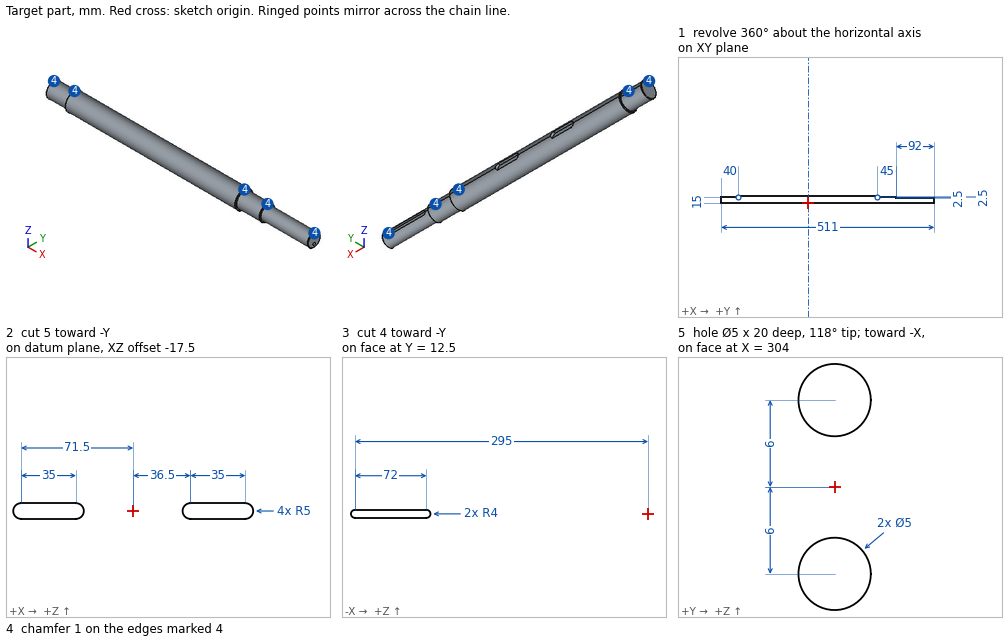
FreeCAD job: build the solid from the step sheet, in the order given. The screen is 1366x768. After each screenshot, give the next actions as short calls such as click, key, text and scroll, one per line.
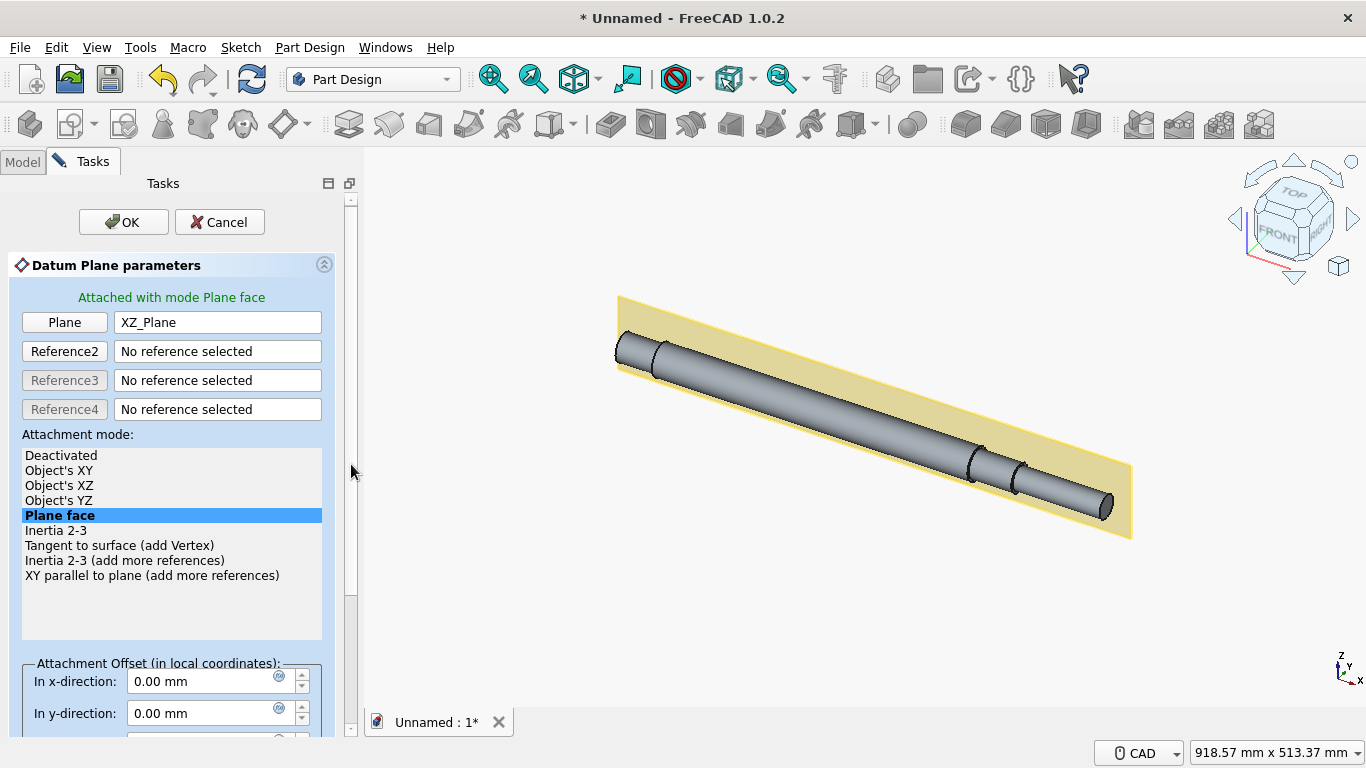
click(124, 222)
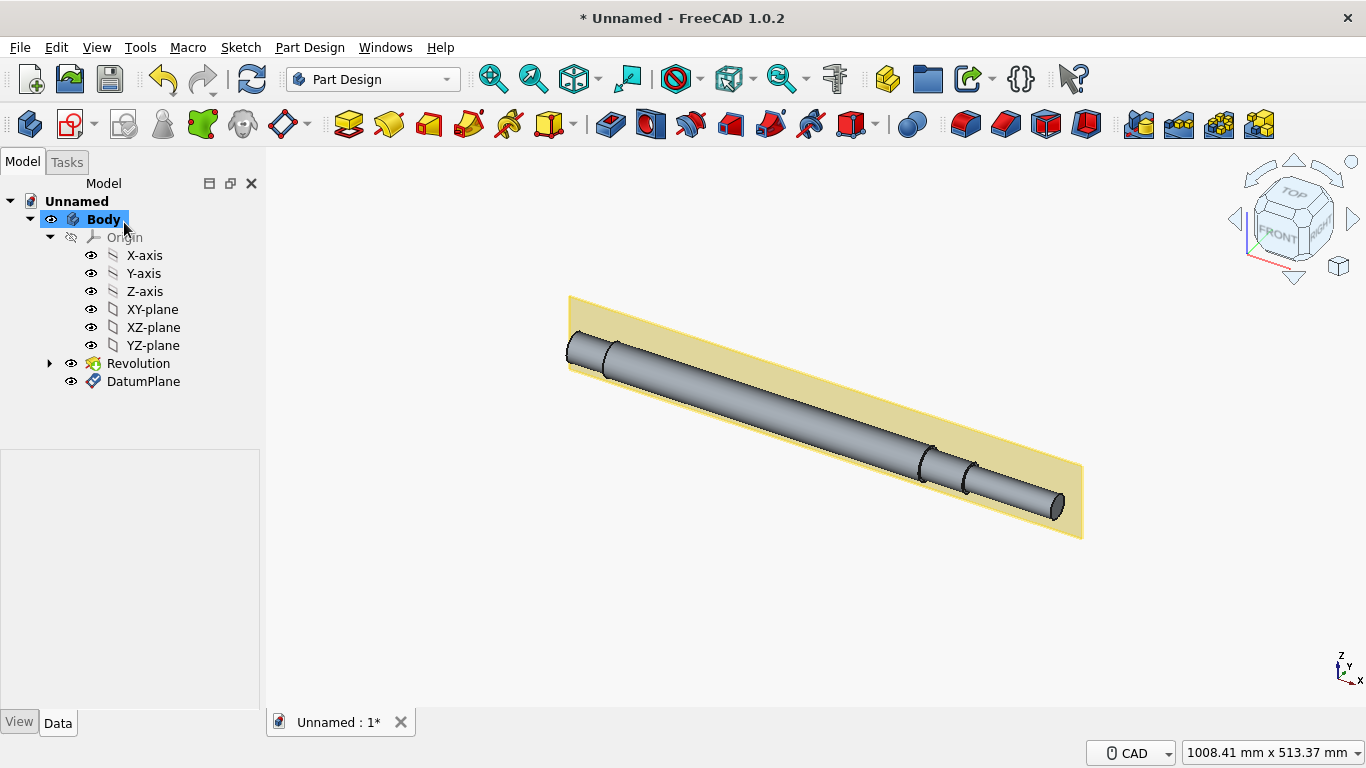
click(116, 381)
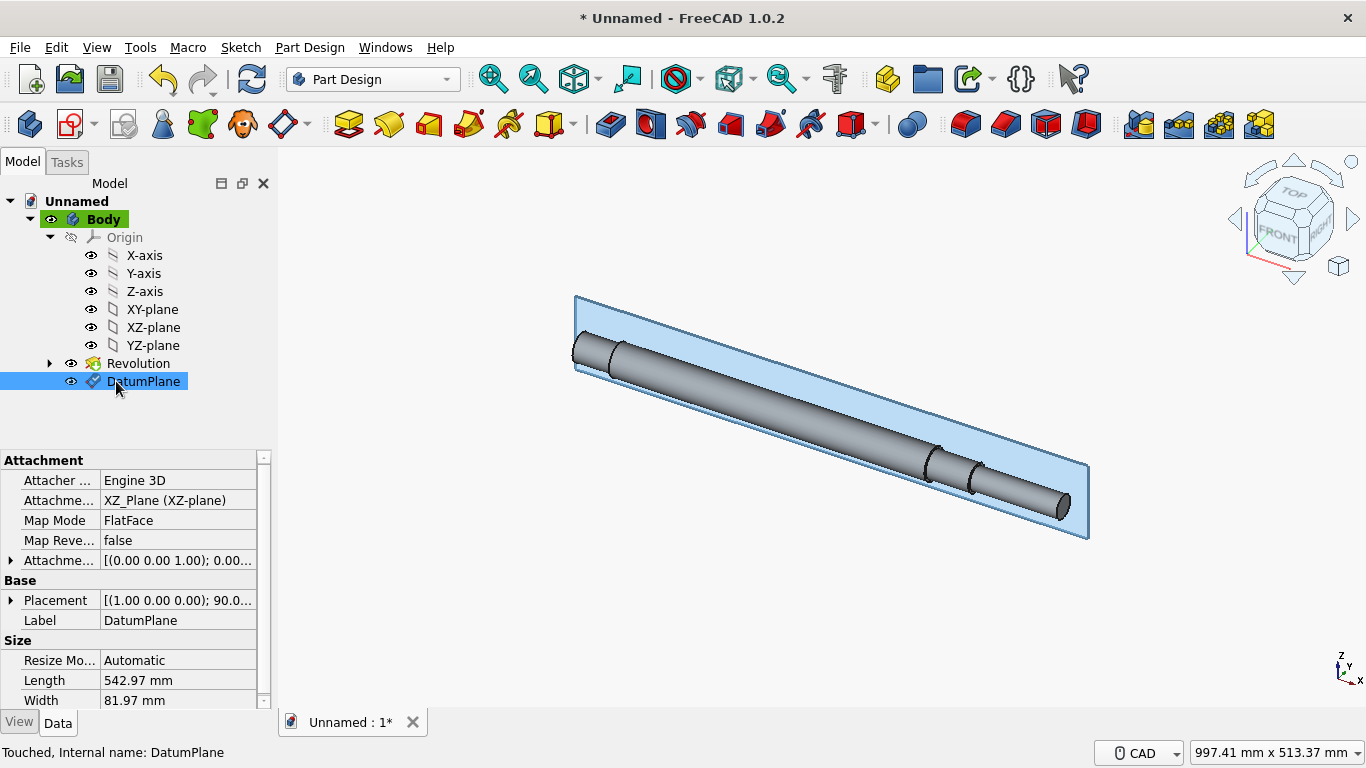
click(70, 124)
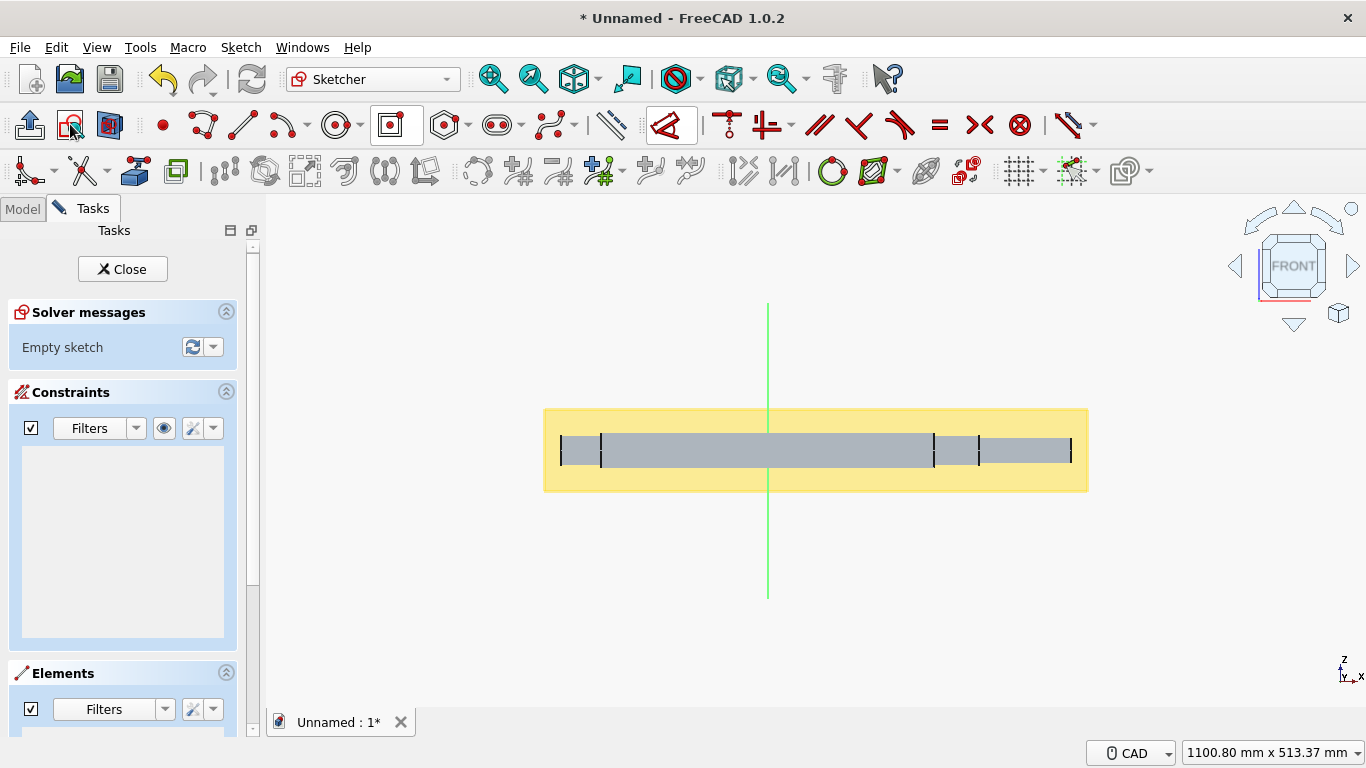
click(110, 126)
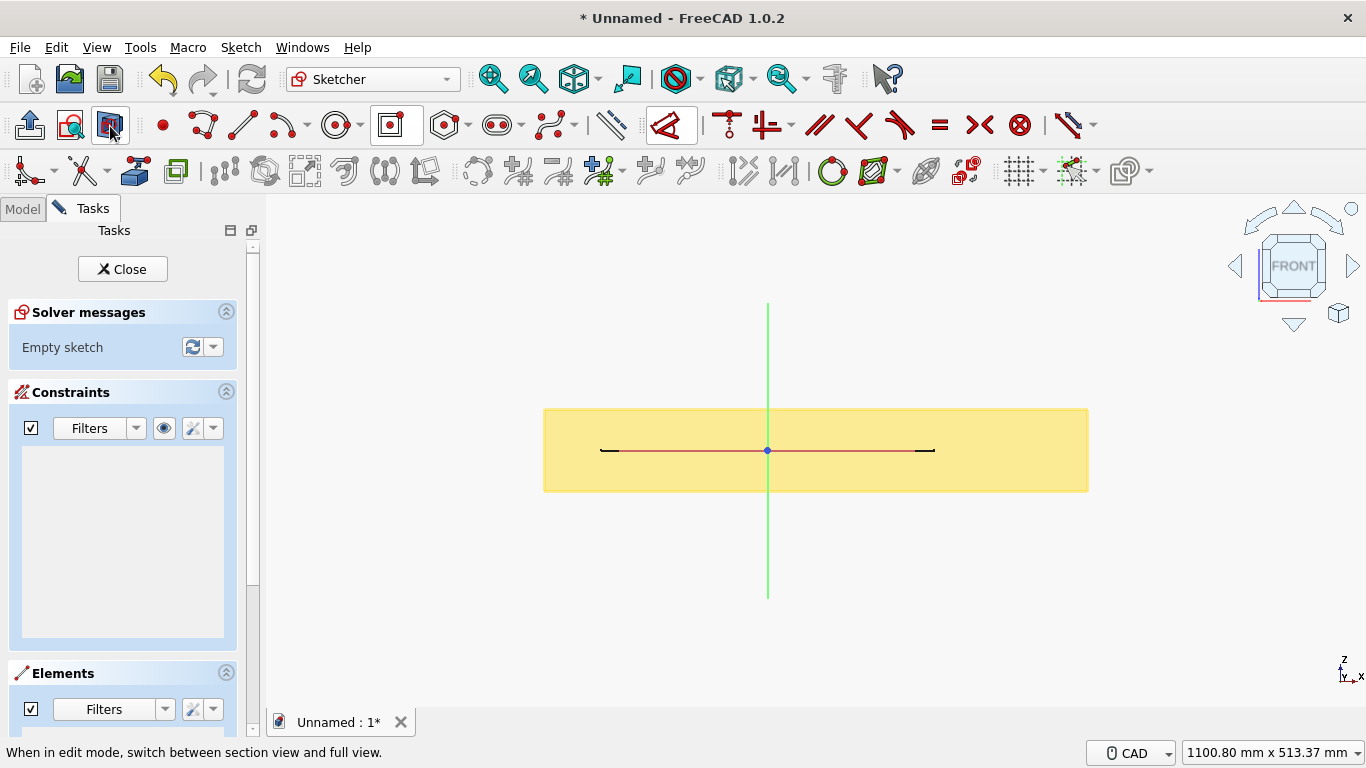
scroll(774, 450, up, 7)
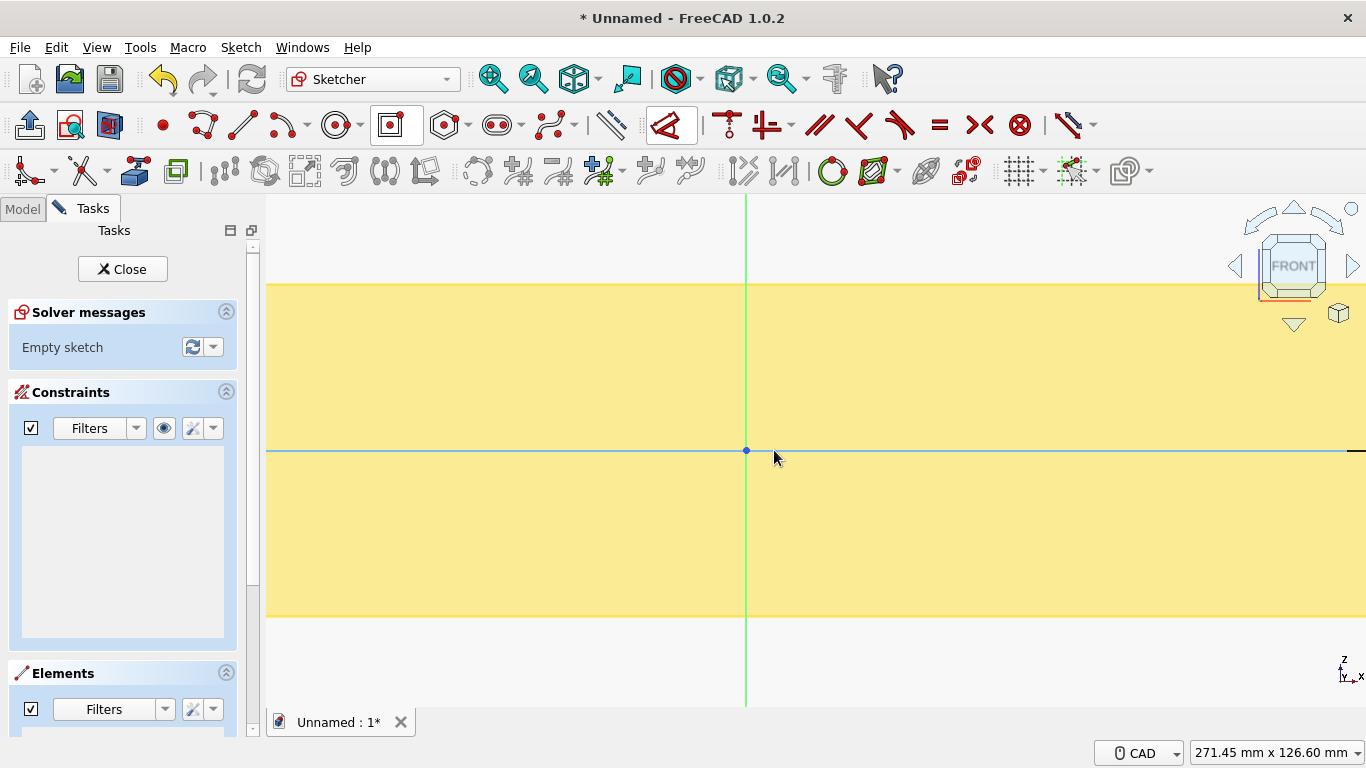
key(g)
key(s)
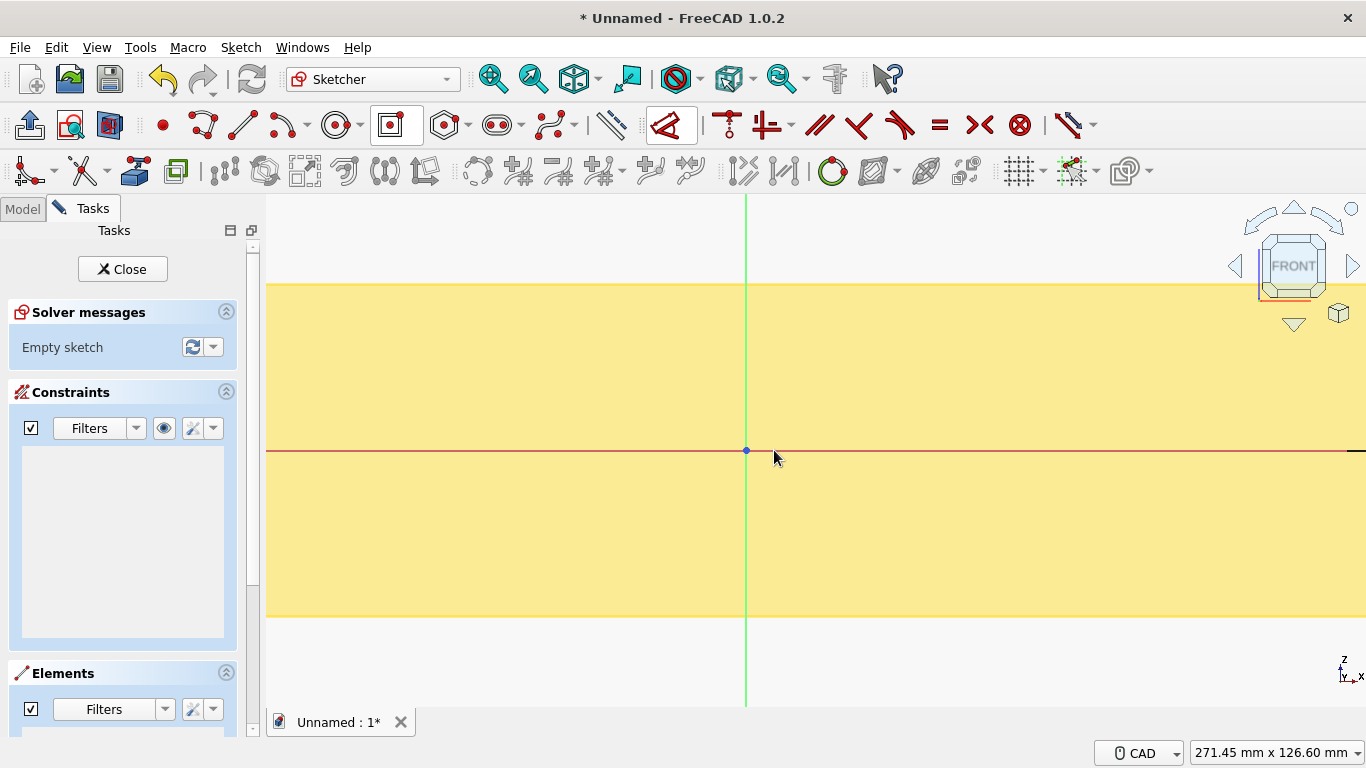
click(894, 450)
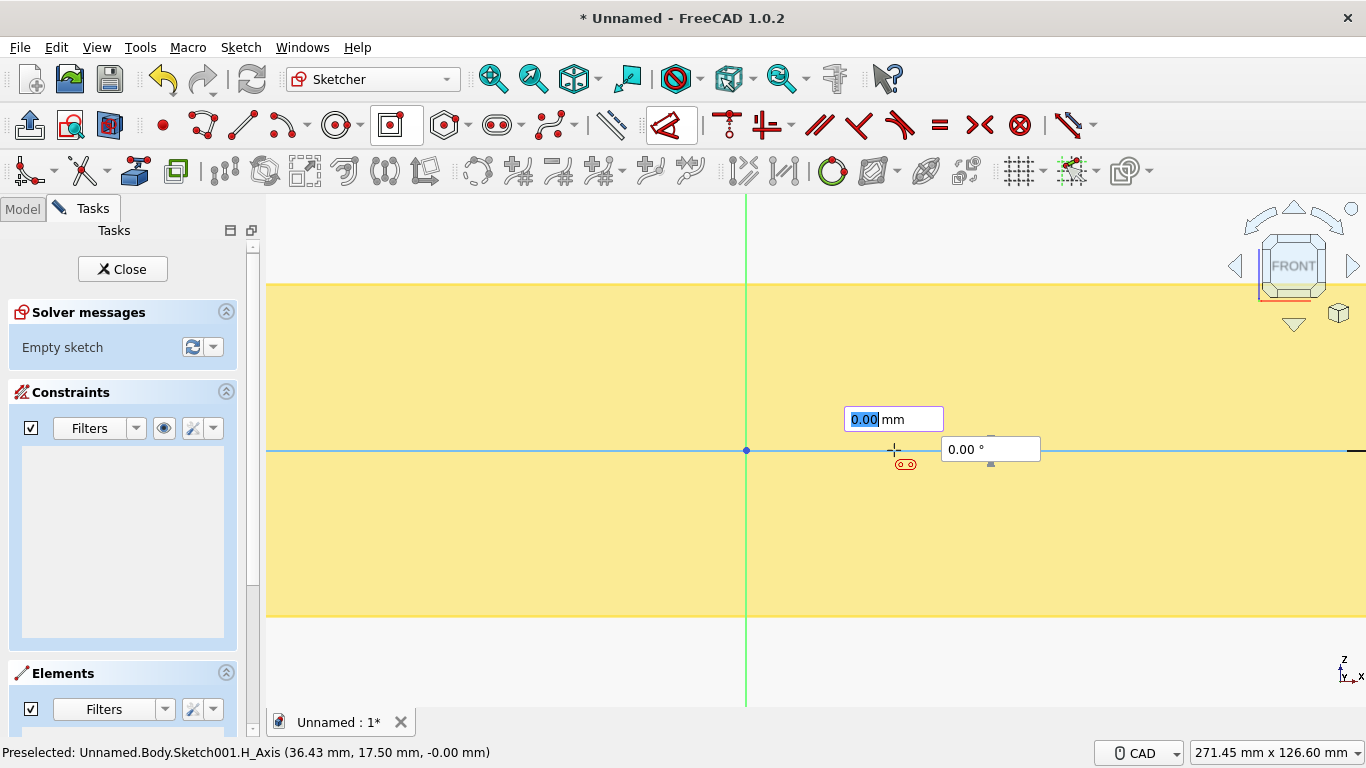
click(1036, 442)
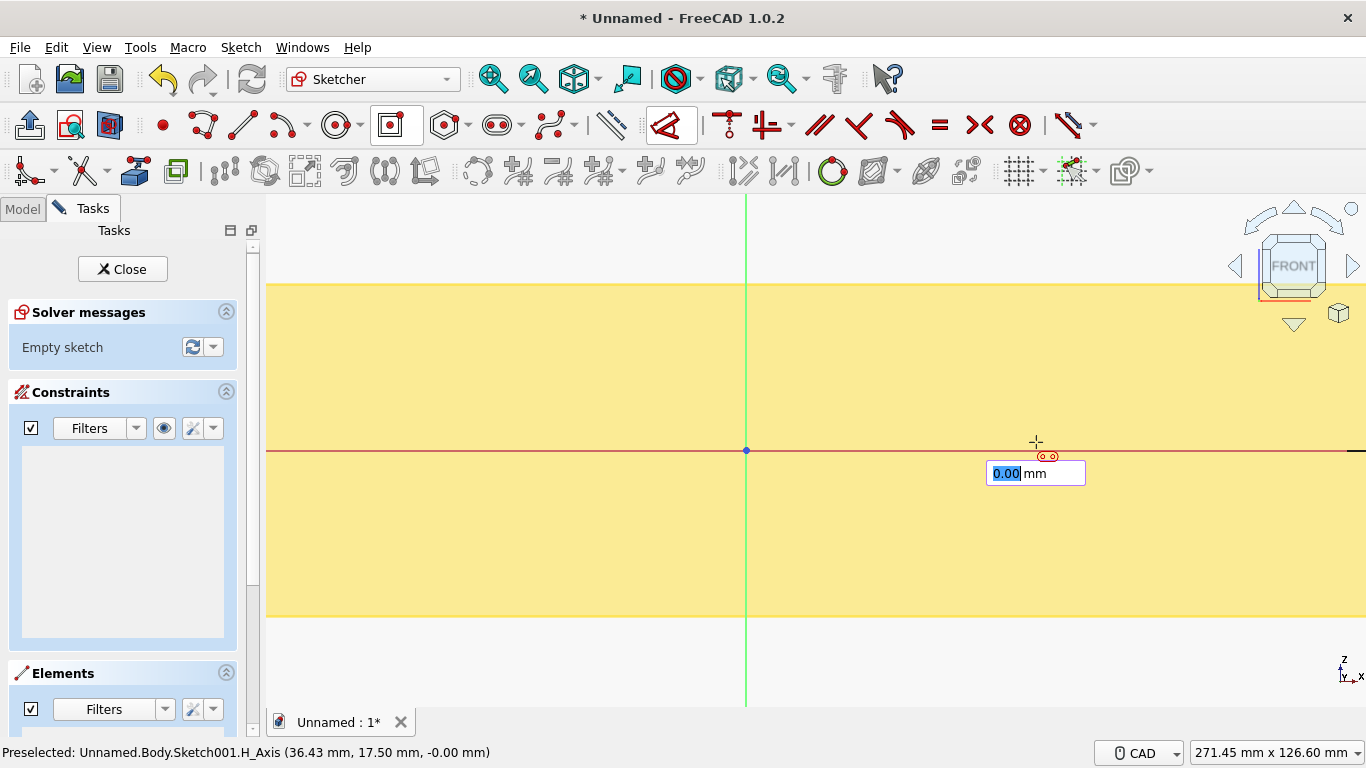
click(965, 471)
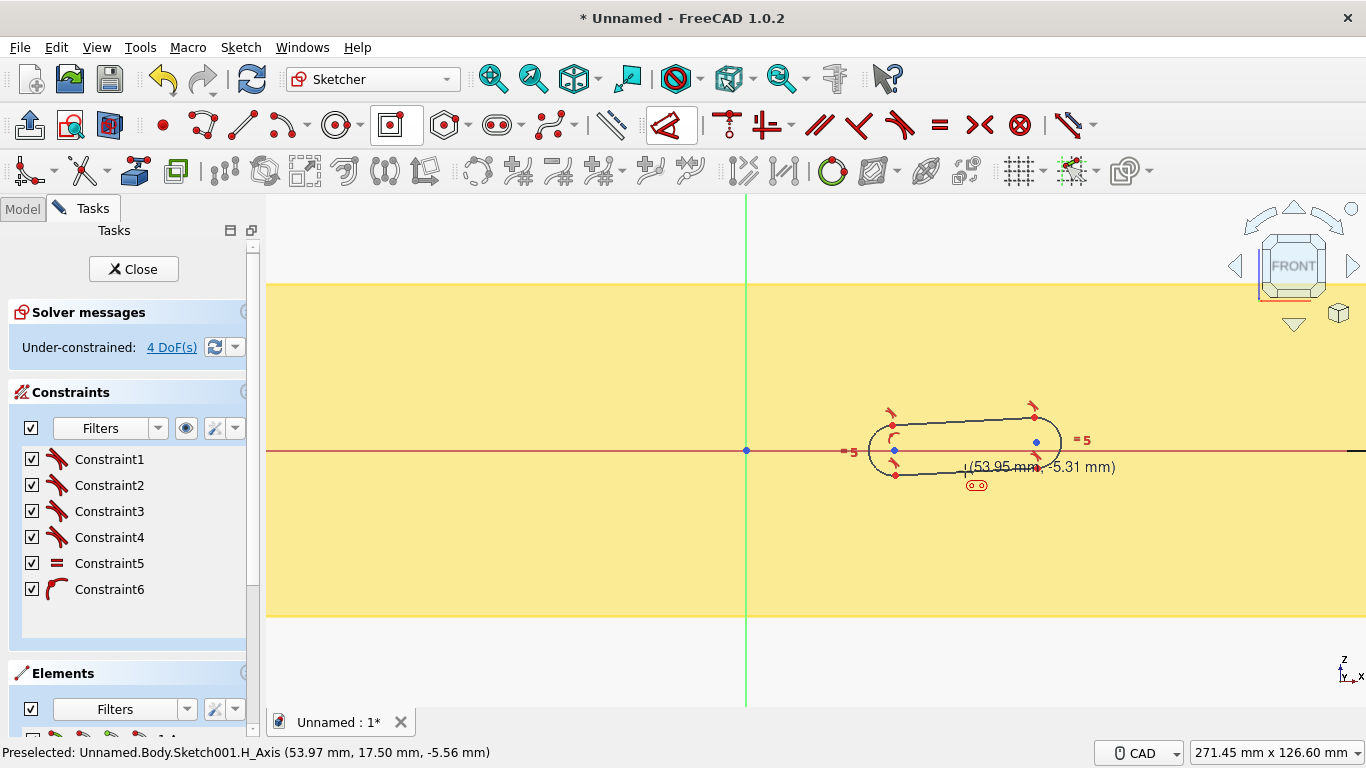
click(457, 450)